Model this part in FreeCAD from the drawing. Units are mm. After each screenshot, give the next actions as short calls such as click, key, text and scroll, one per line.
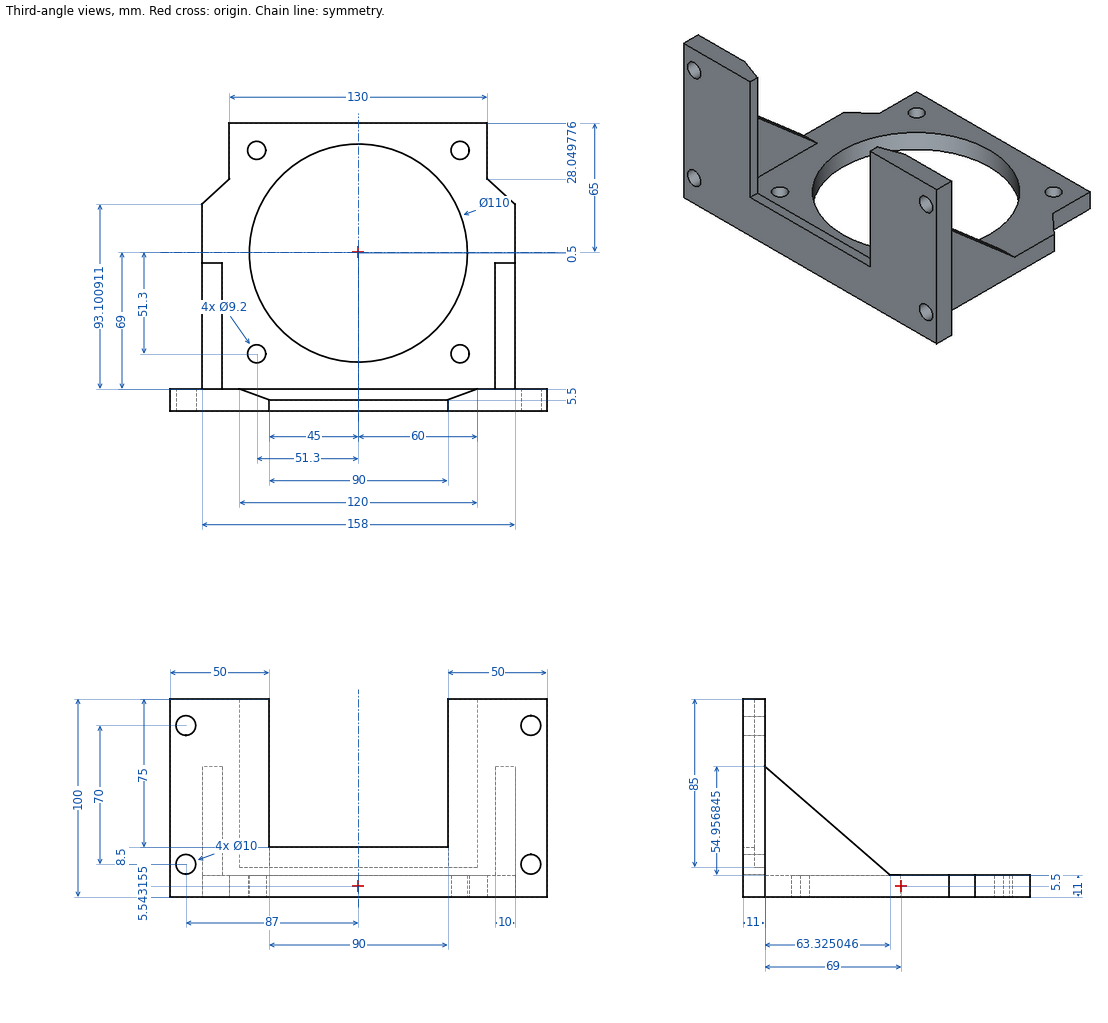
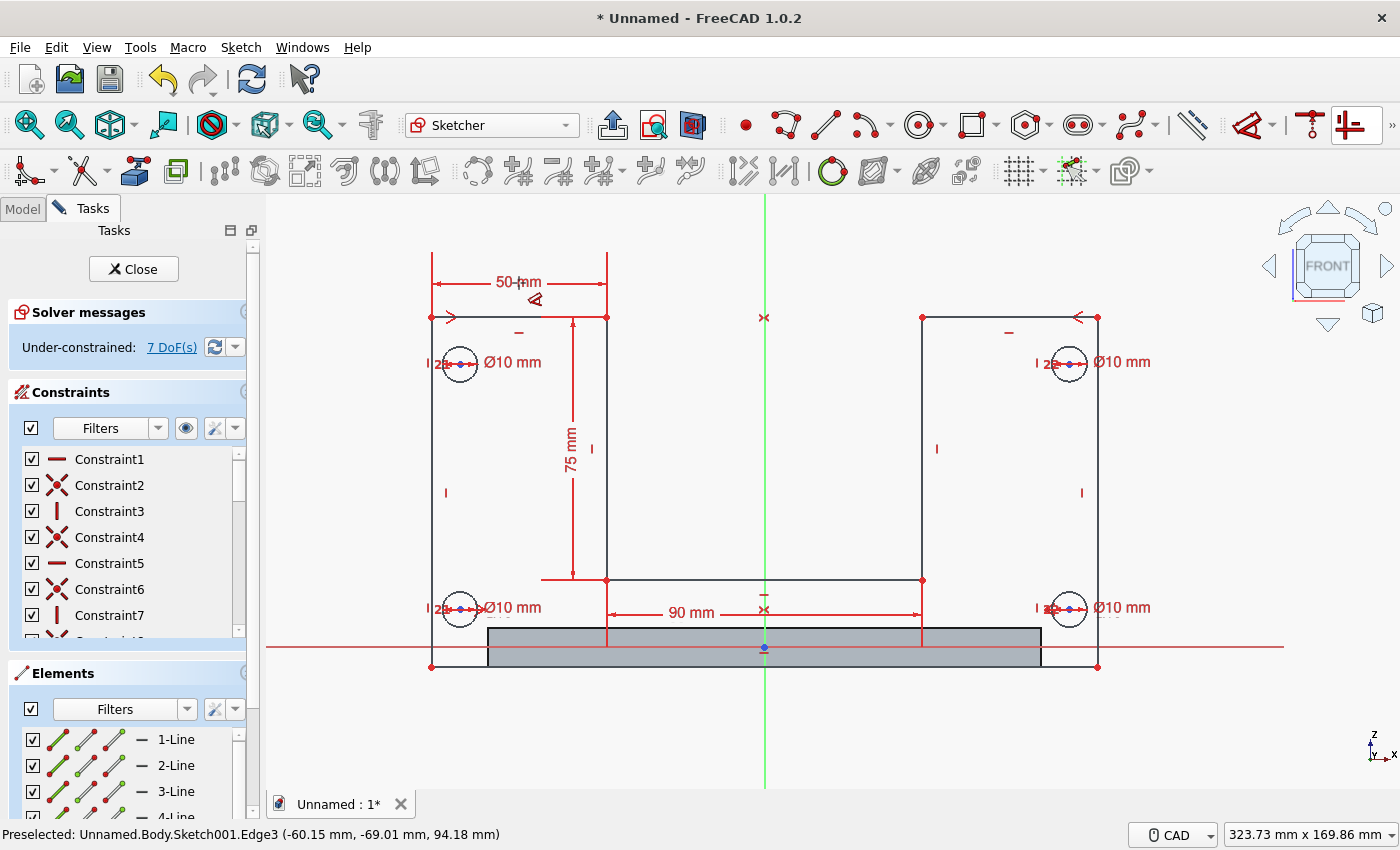
click(1045, 317)
click(1010, 283)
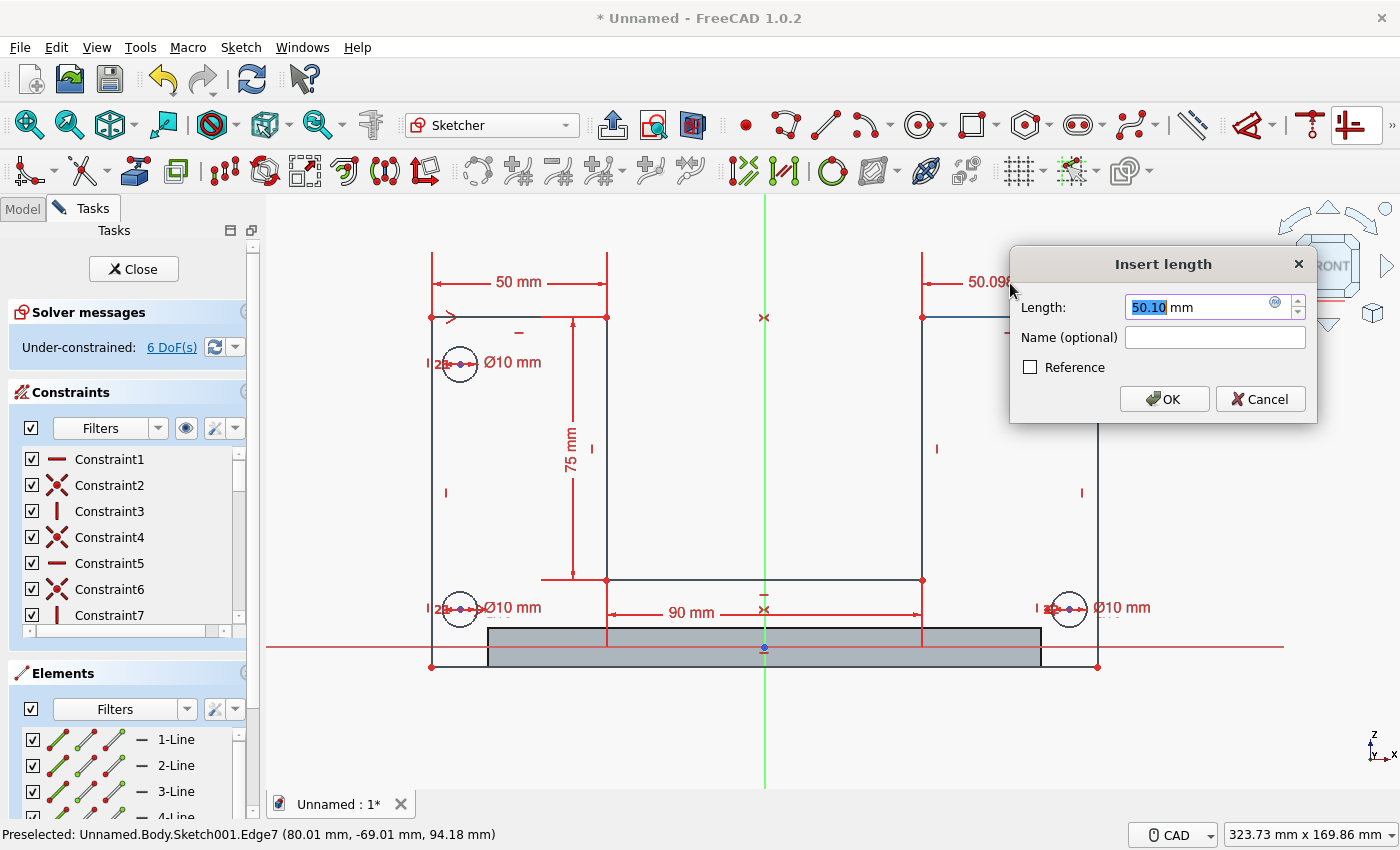
text(50)
key(Return)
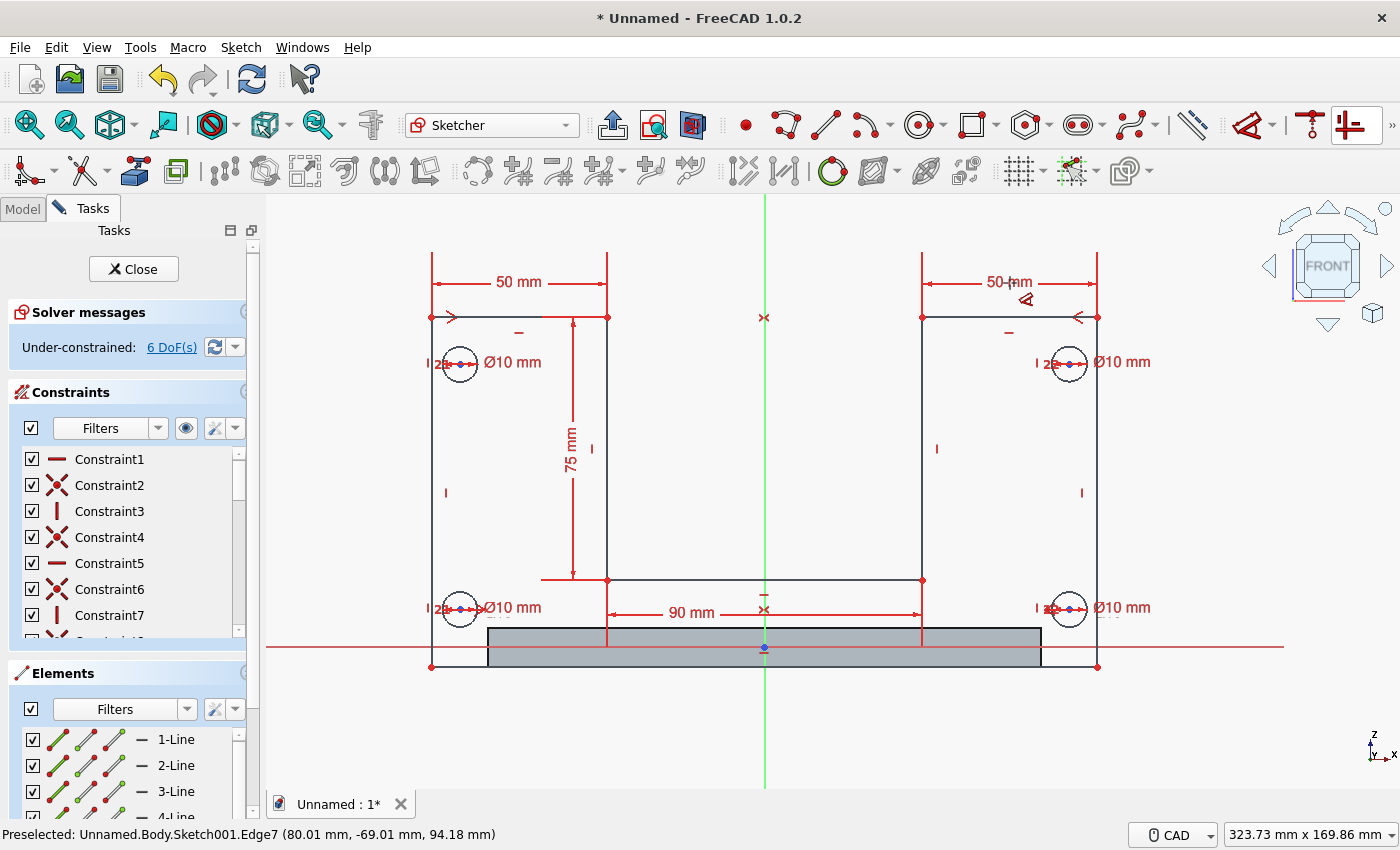
click(460, 610)
click(612, 681)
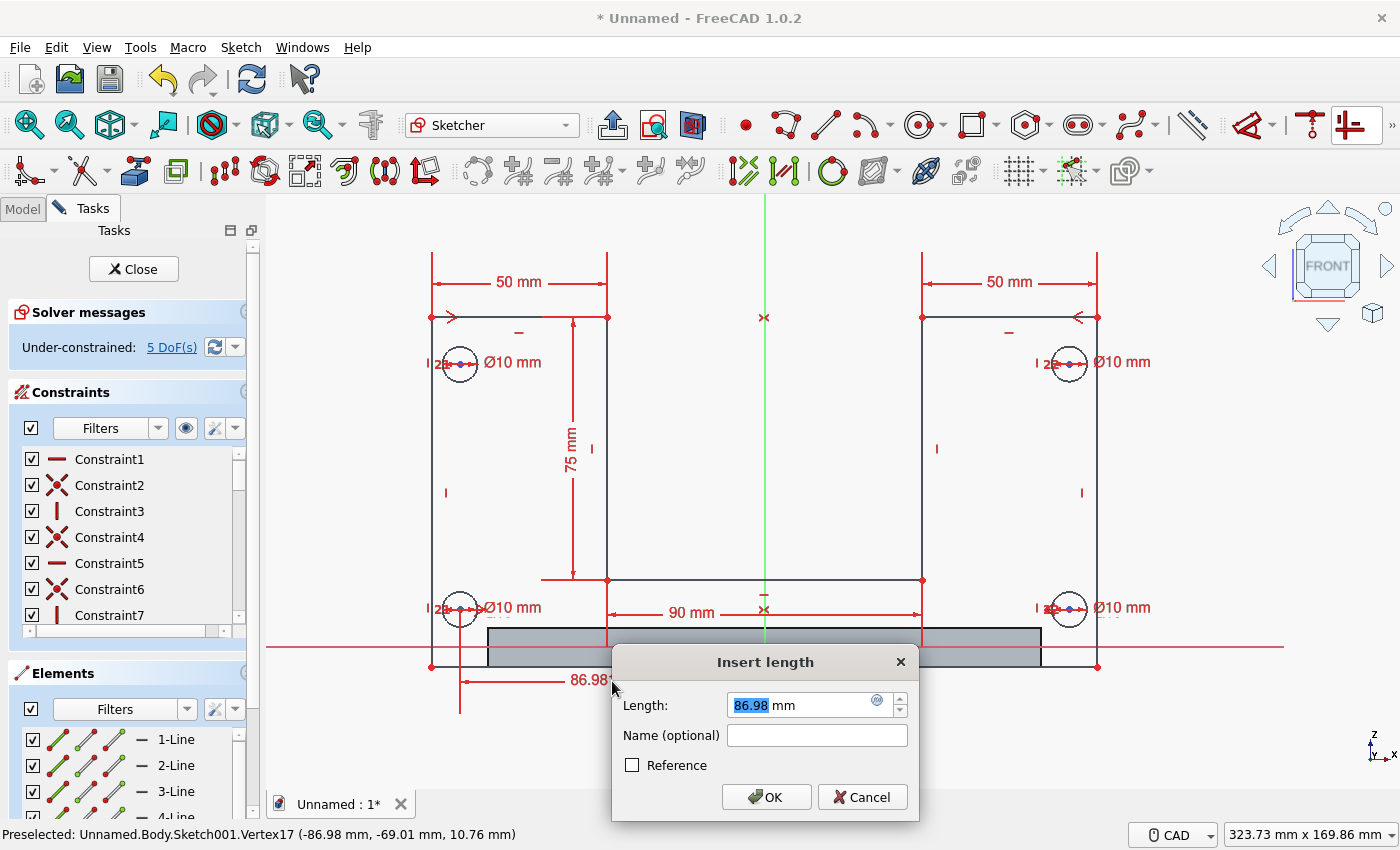
text(87)
key(Return)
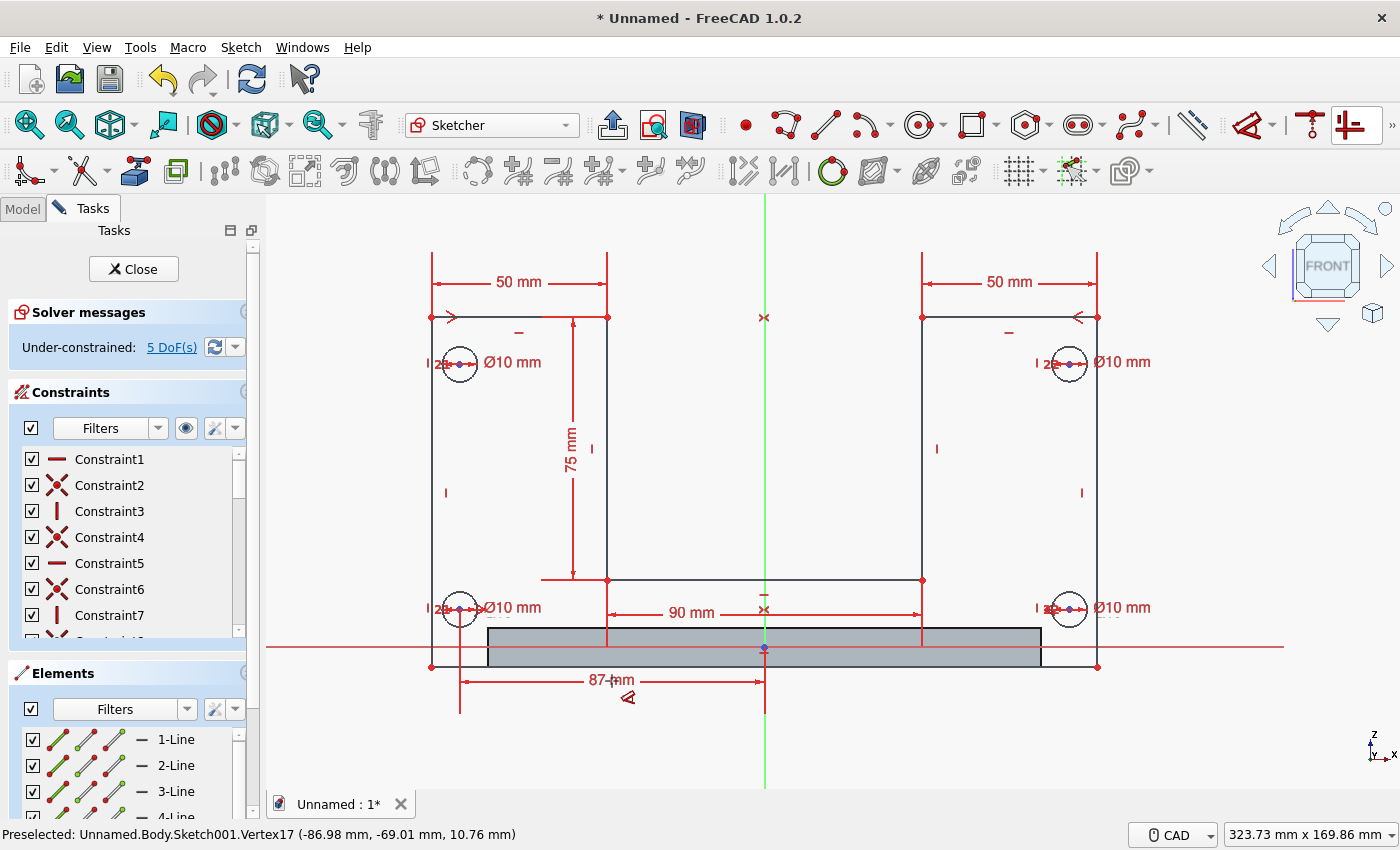
click(432, 422)
click(398, 492)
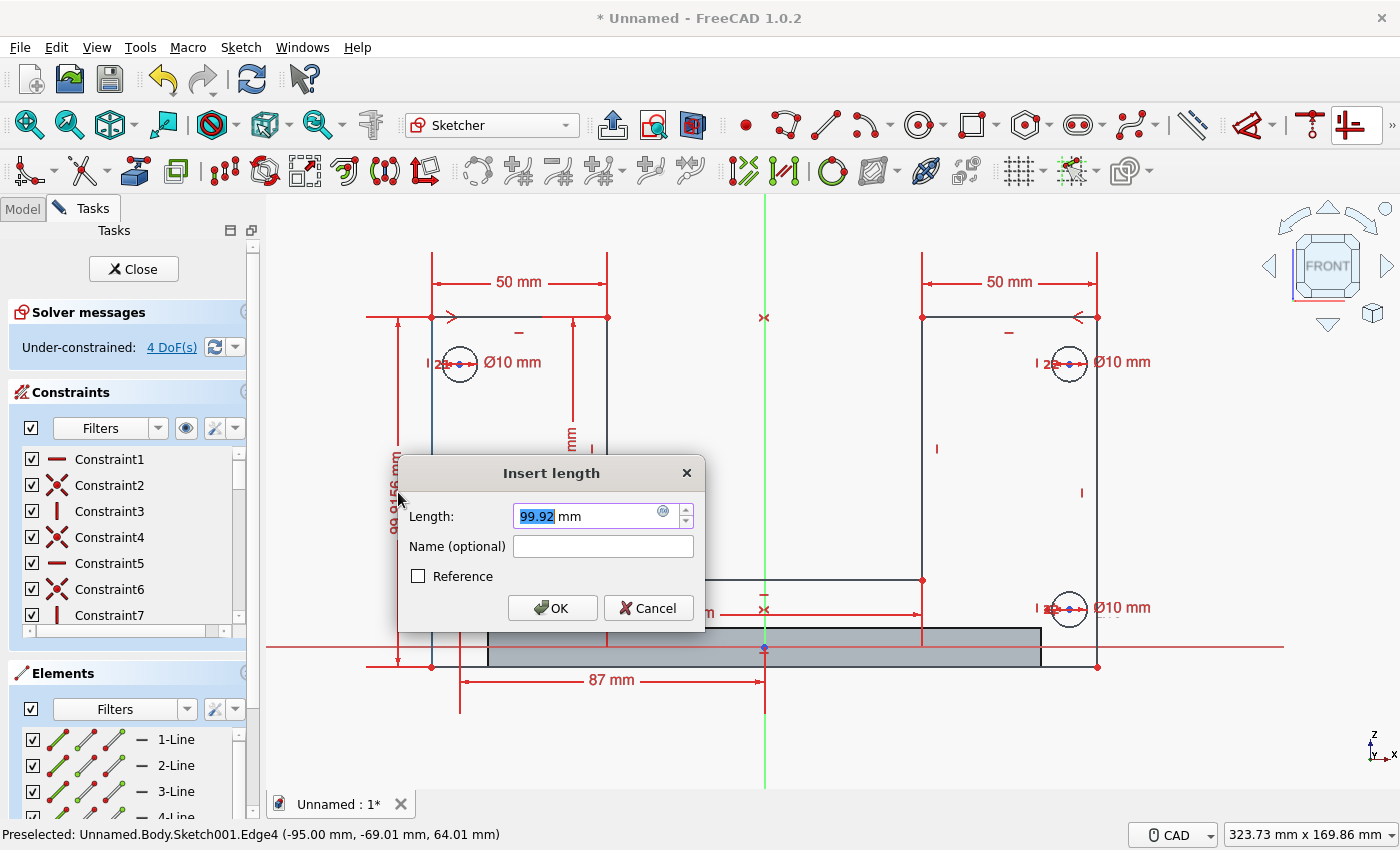
text(100)
key(Return)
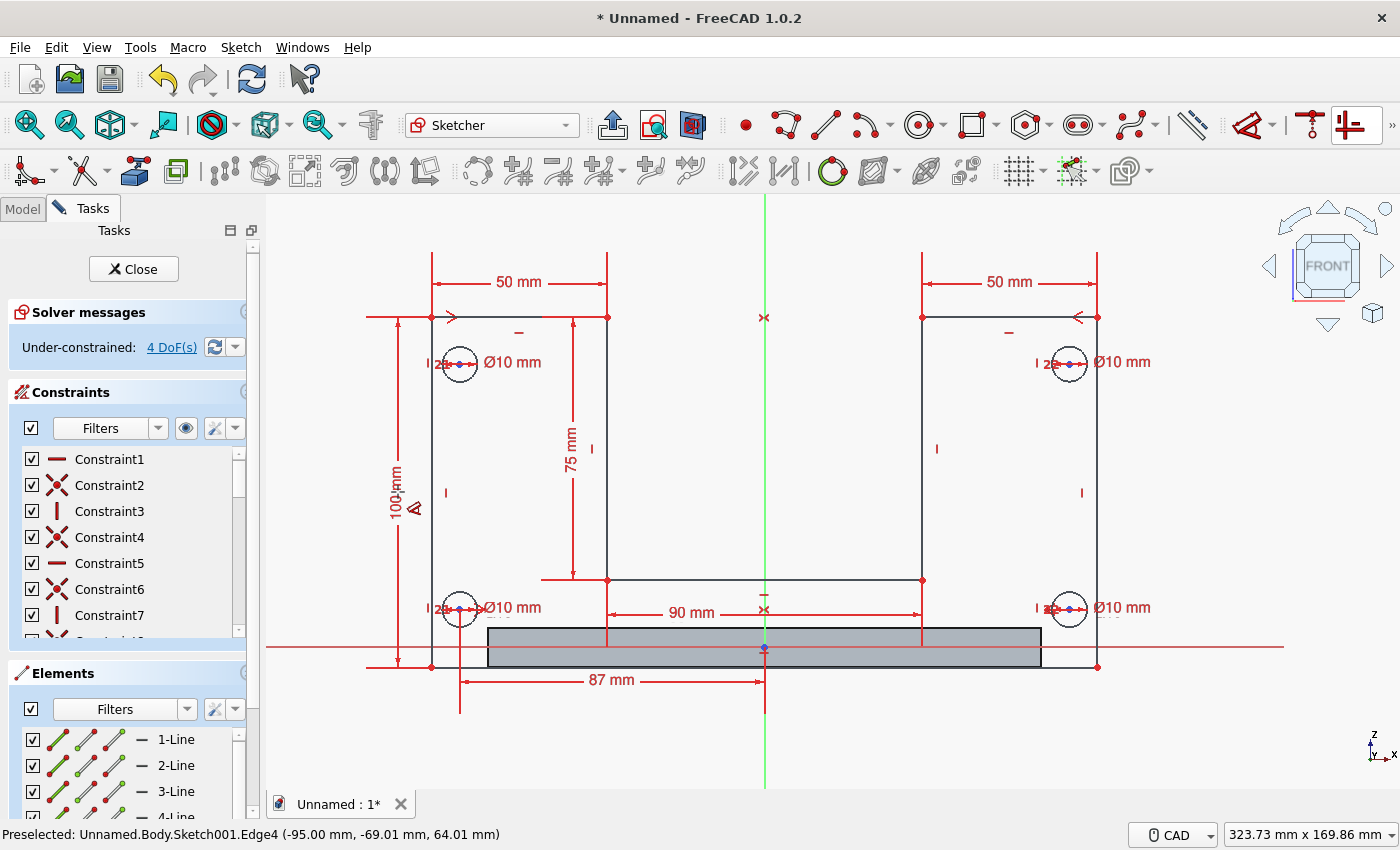
click(460, 610)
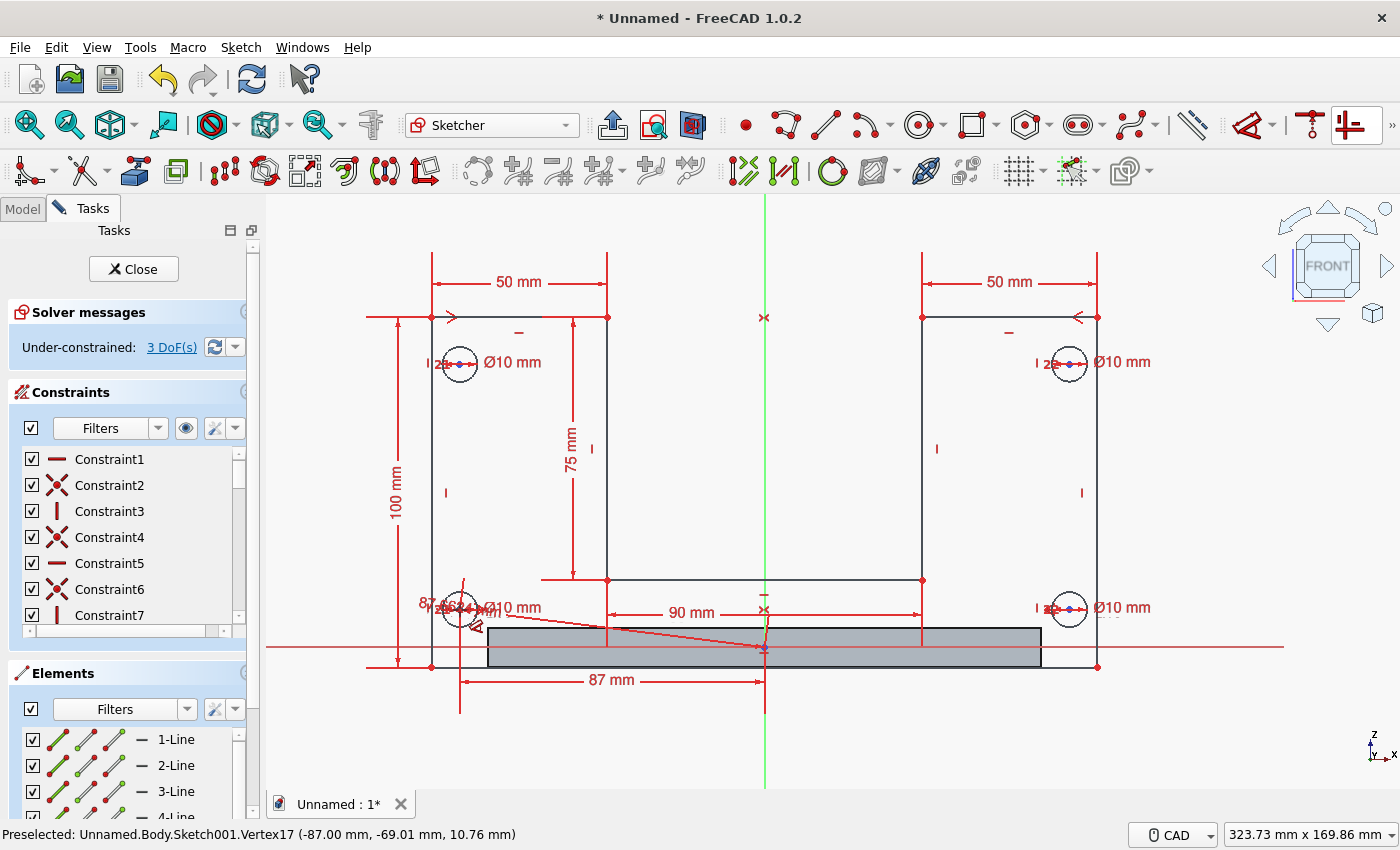
click(460, 364)
click(494, 487)